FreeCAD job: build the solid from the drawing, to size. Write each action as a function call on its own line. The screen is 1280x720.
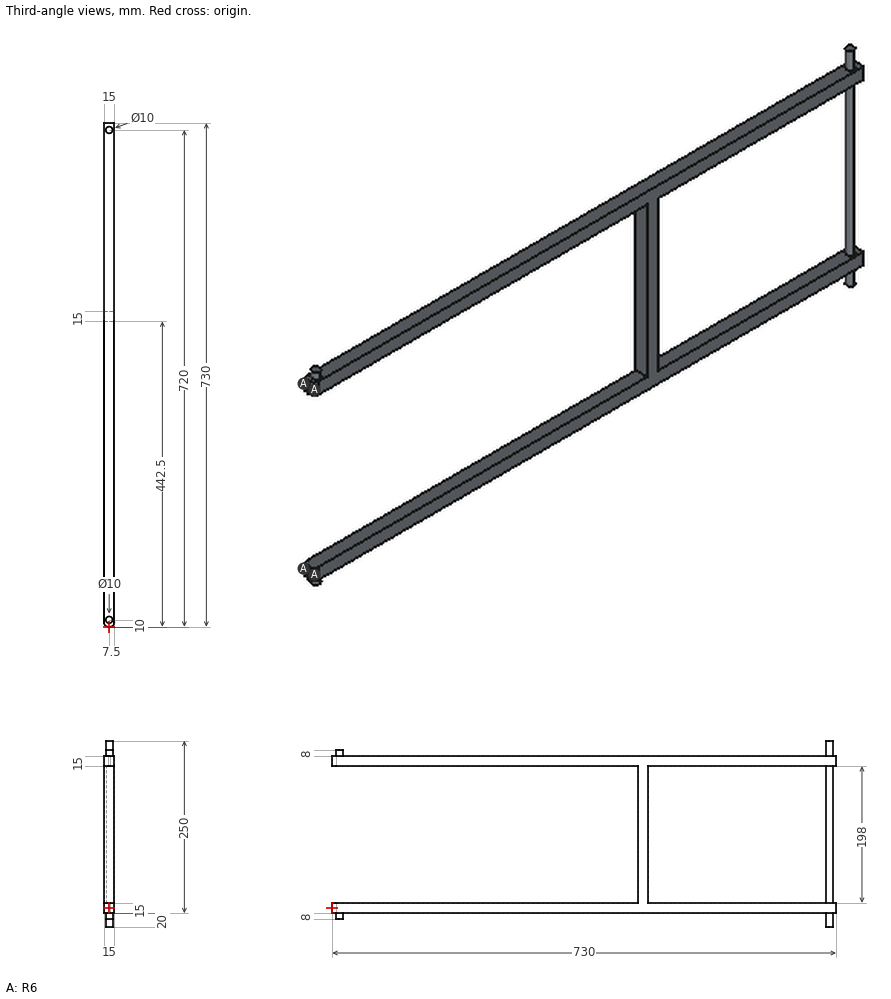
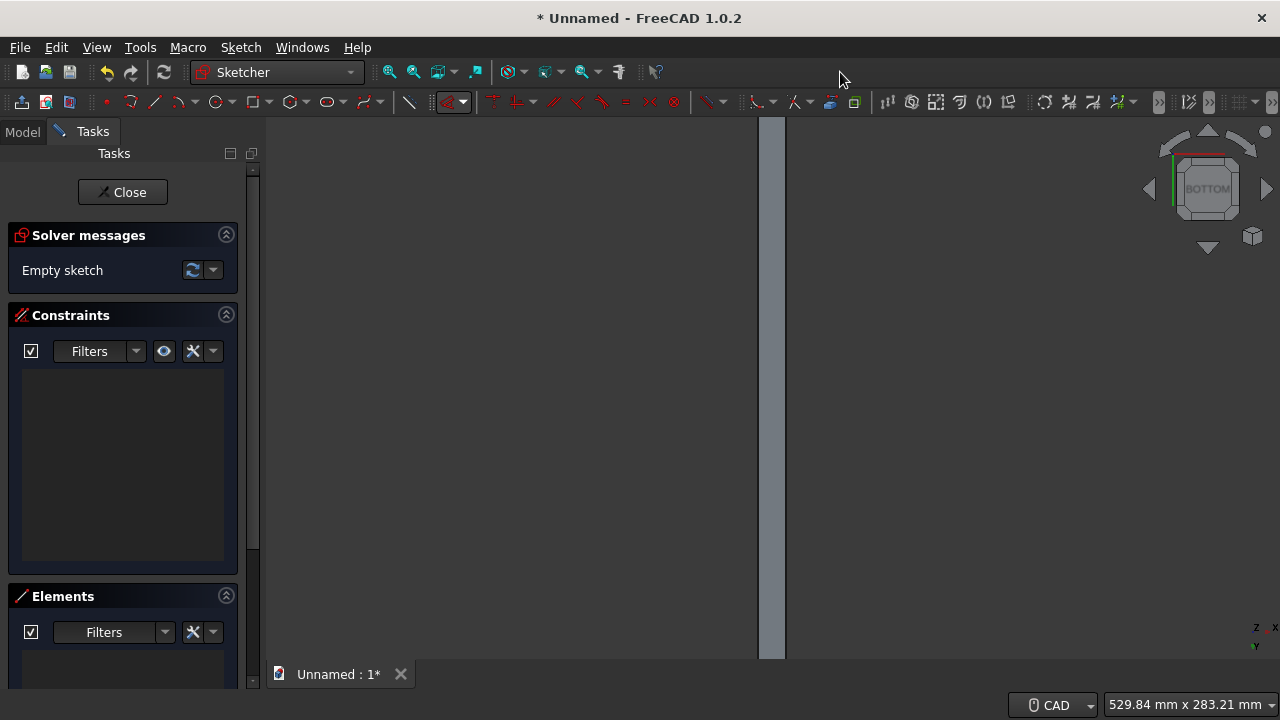
click(70, 102)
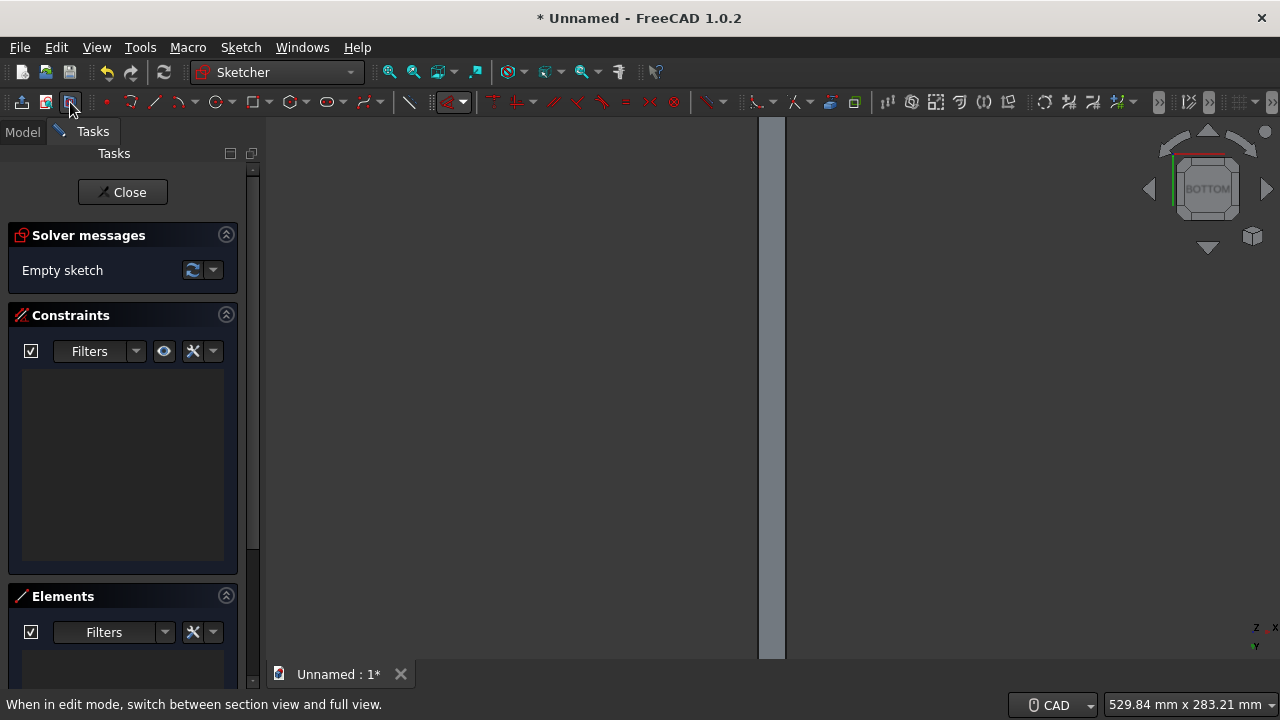
scroll(704, 388, down, 5)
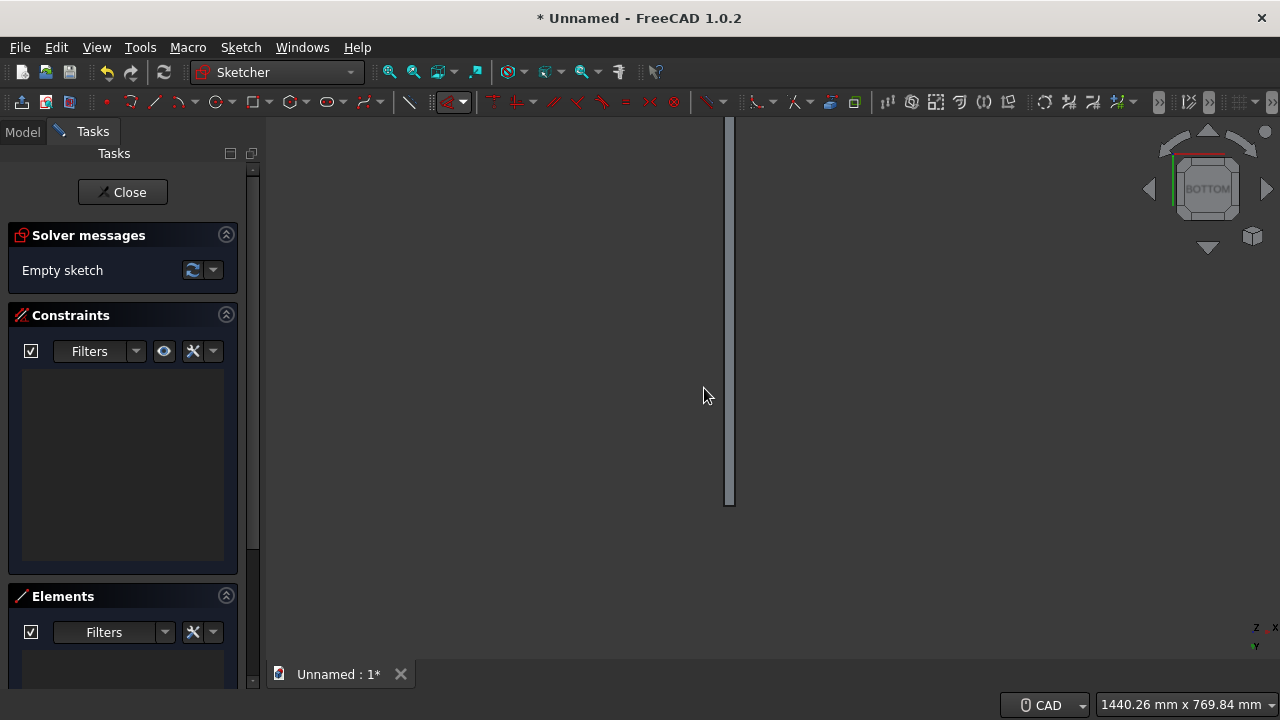
scroll(731, 505, up, 15)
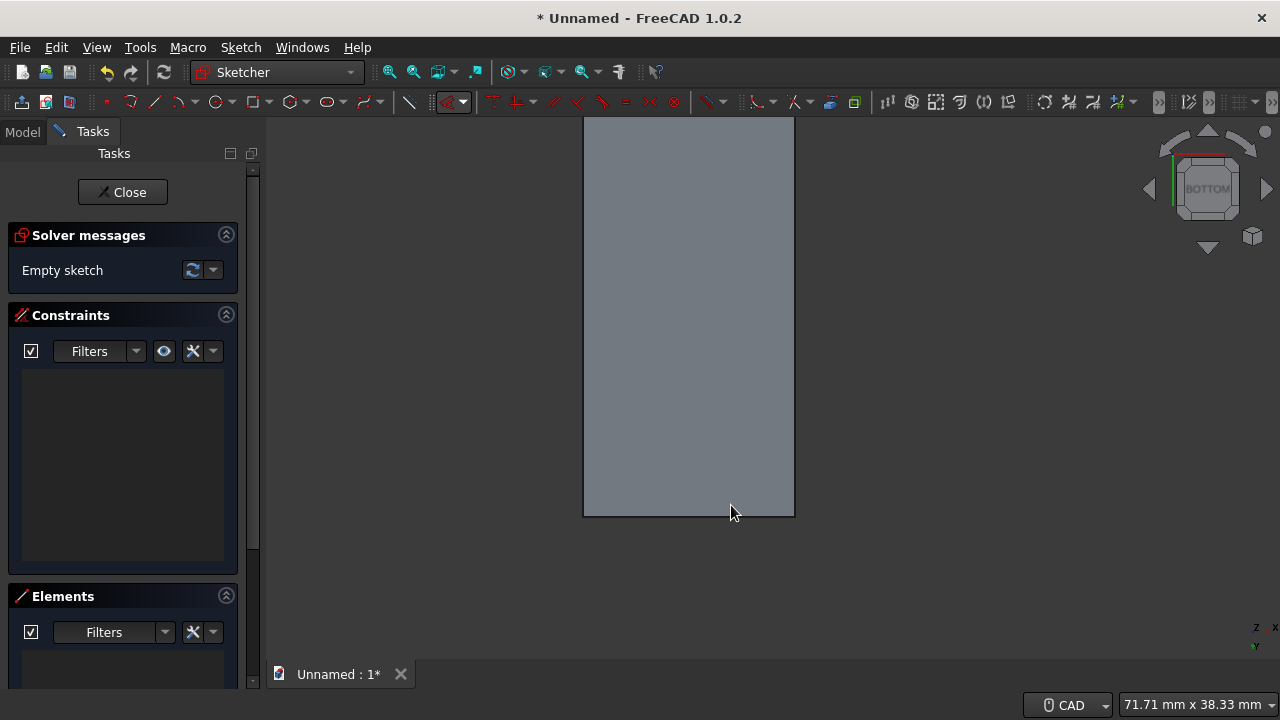
scroll(676, 366, up, 4)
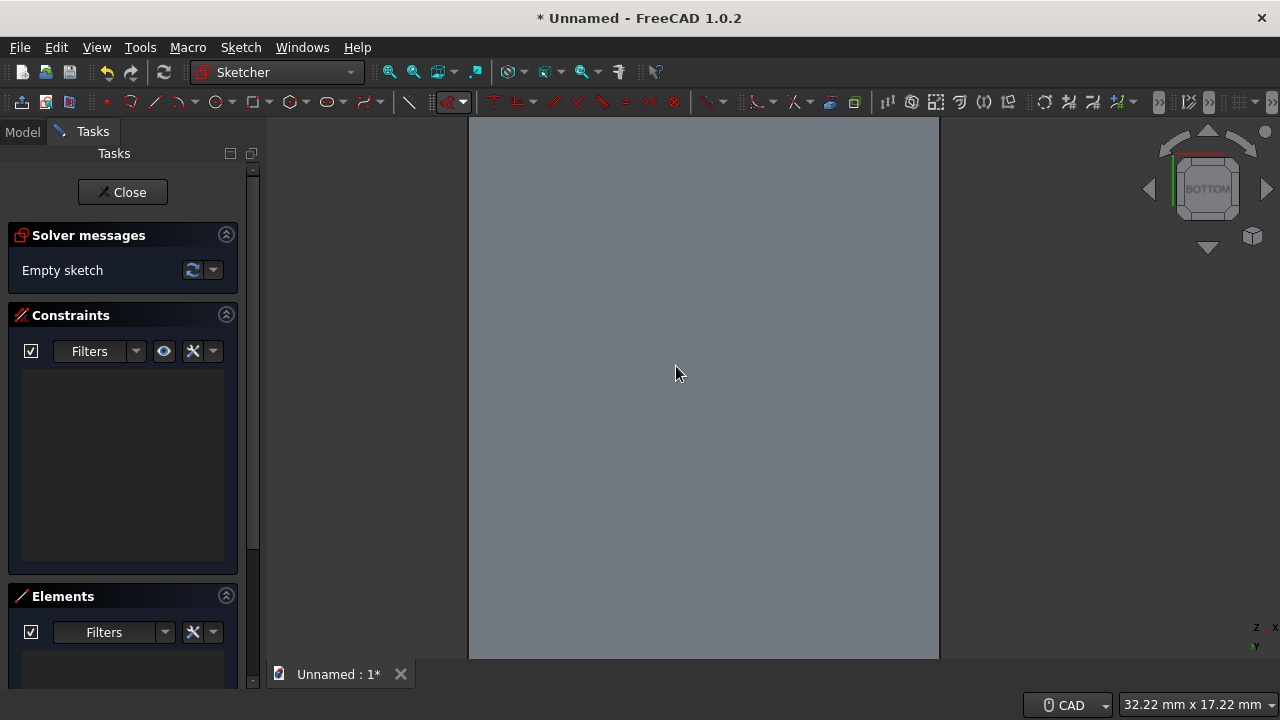
click(216, 102)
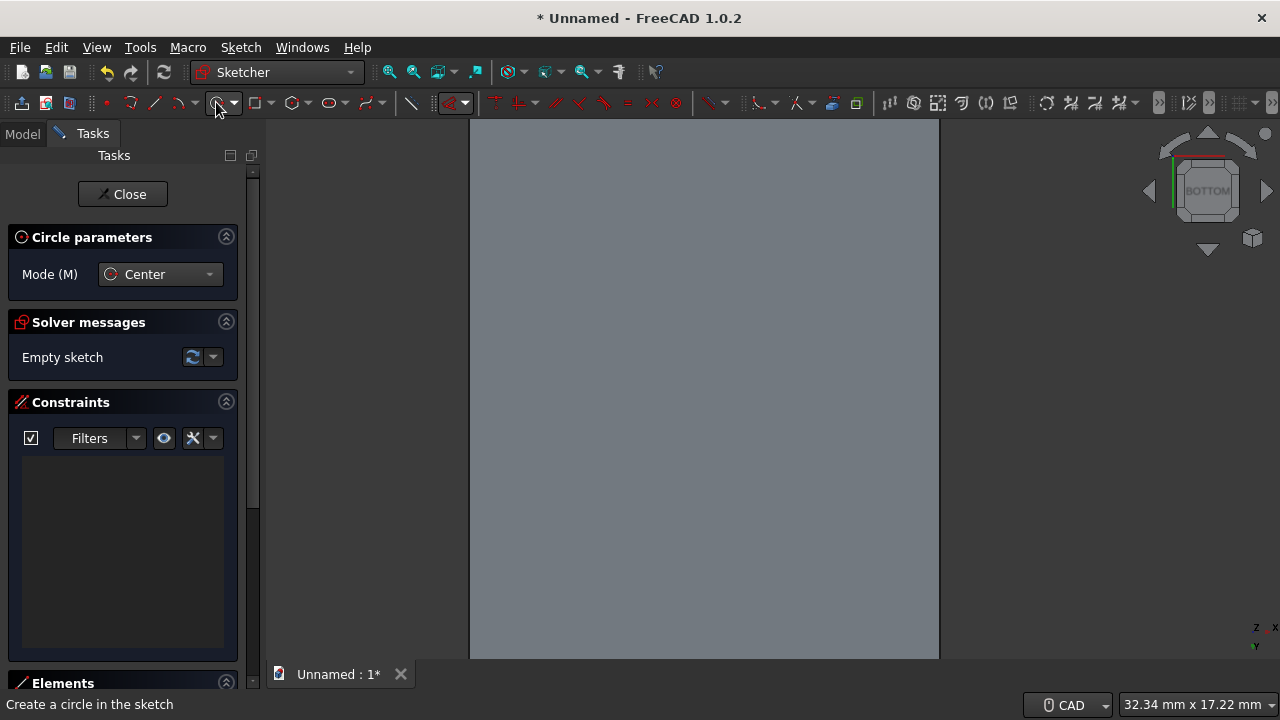
click(704, 388)
move(815, 277)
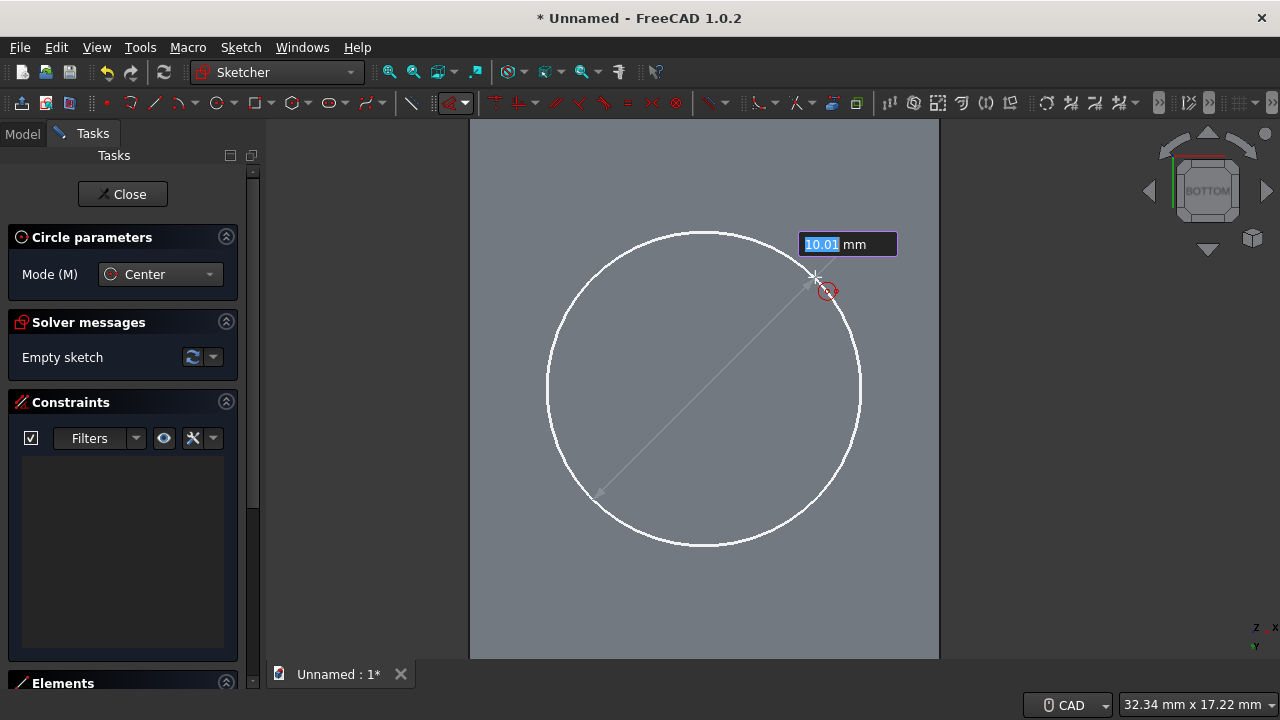
text(10)
key(Return)
key(Escape)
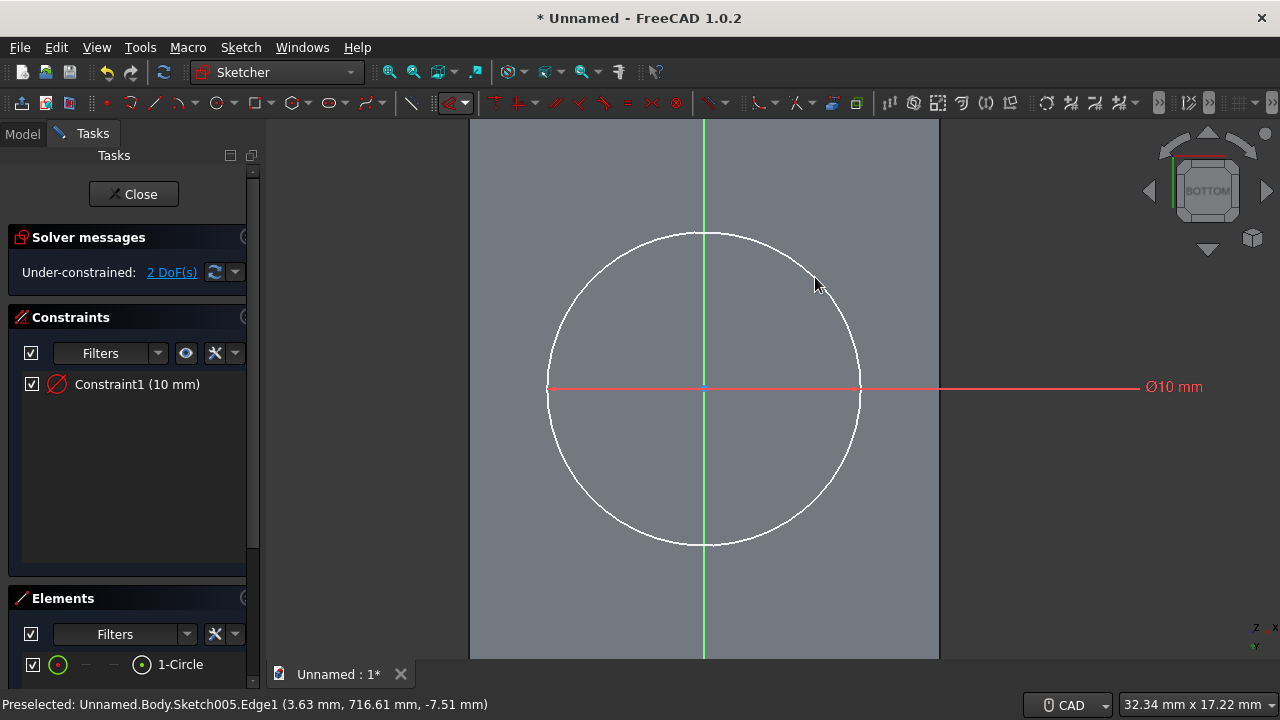
click(704, 389)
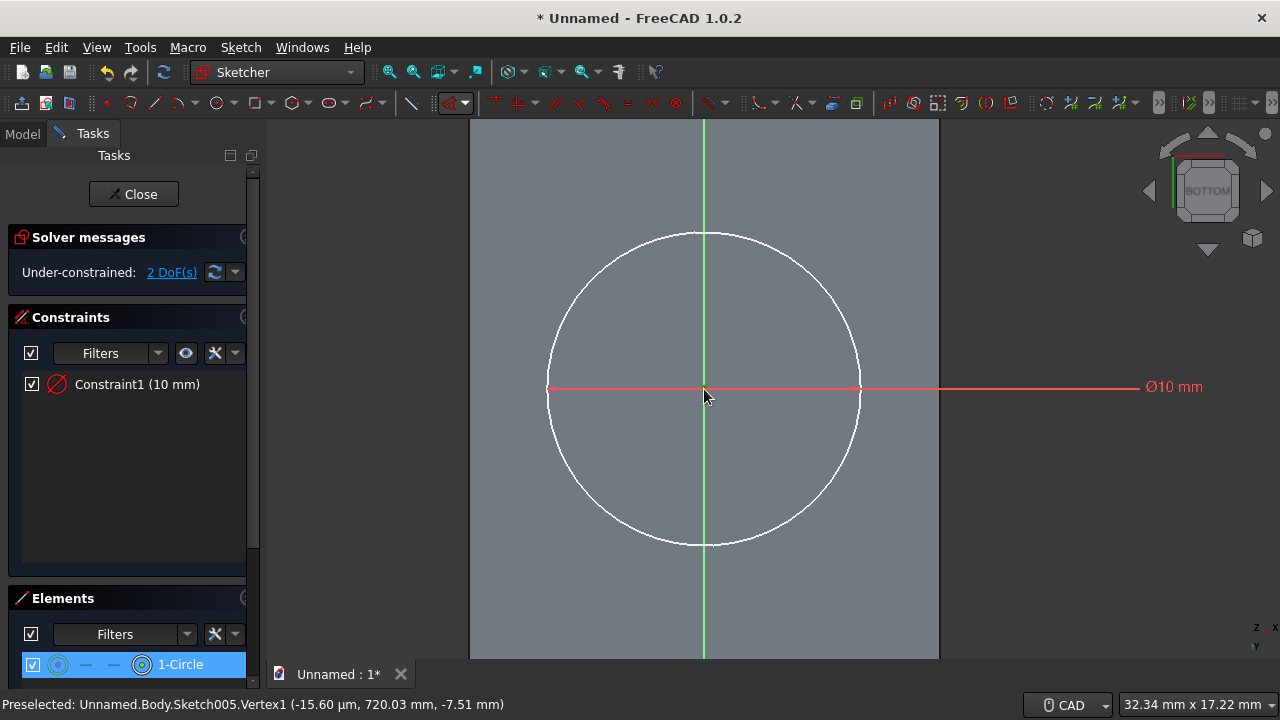
click(704, 596)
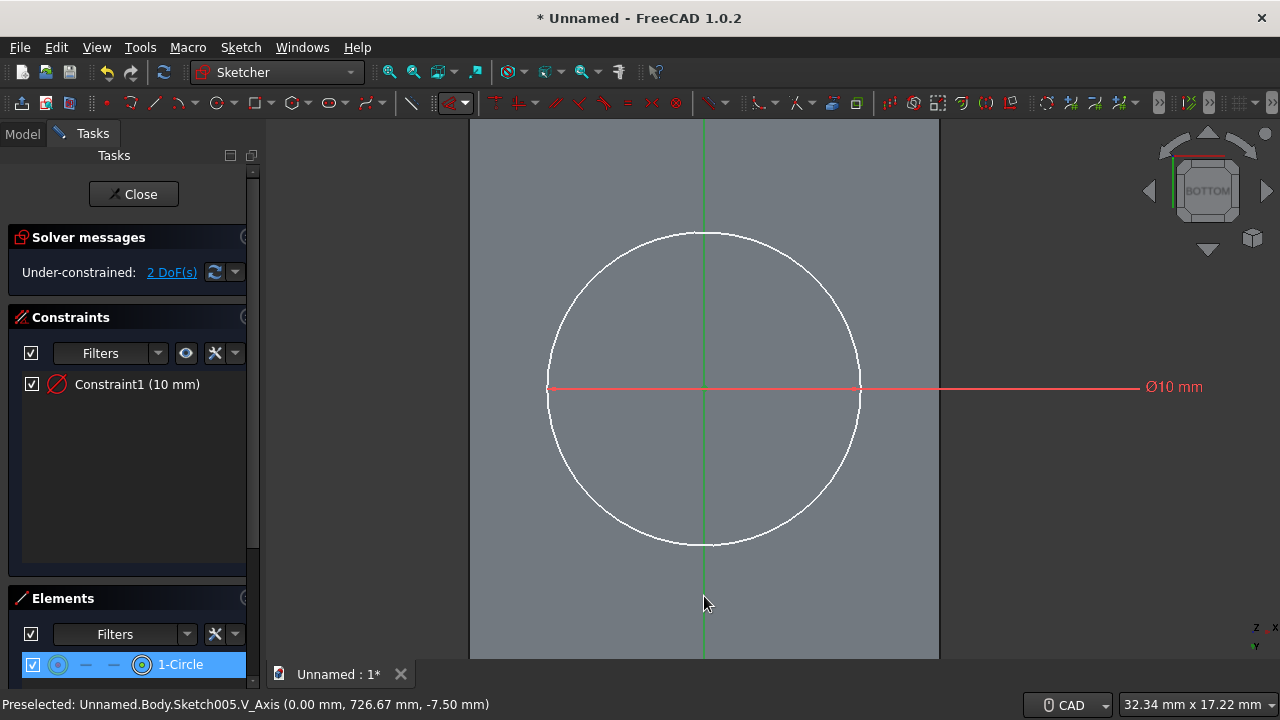
click(496, 104)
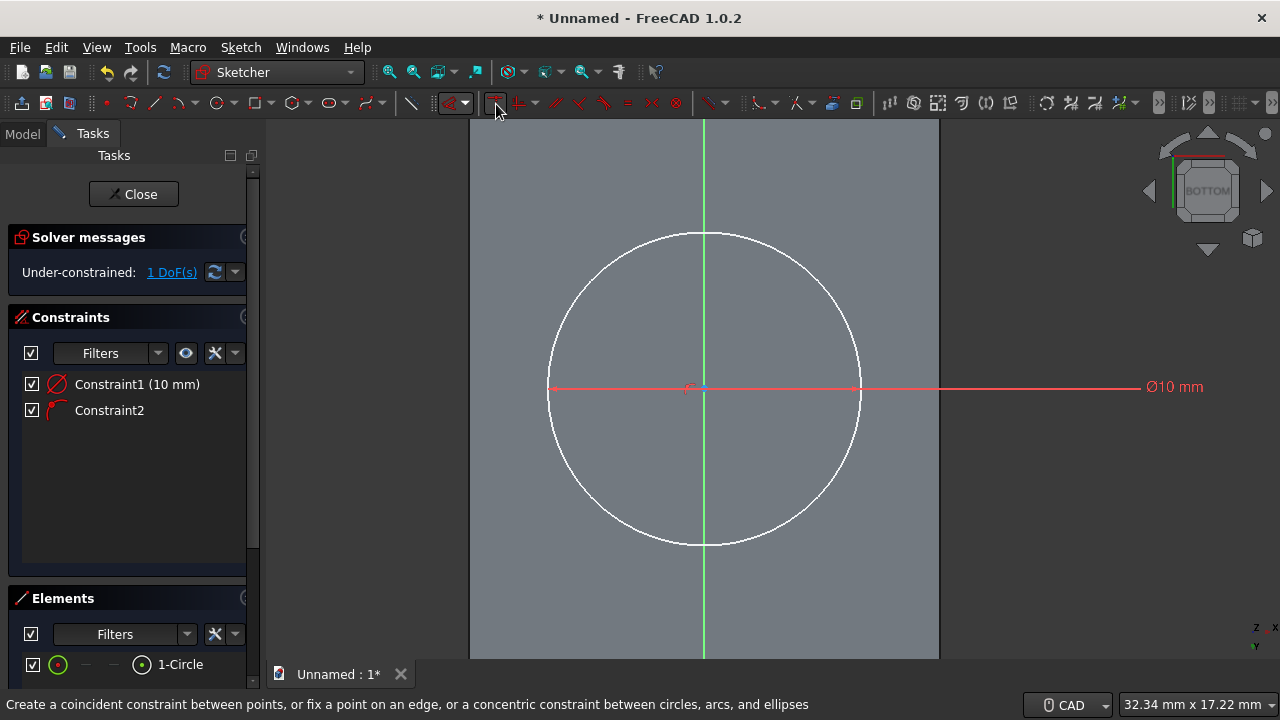
click(704, 389)